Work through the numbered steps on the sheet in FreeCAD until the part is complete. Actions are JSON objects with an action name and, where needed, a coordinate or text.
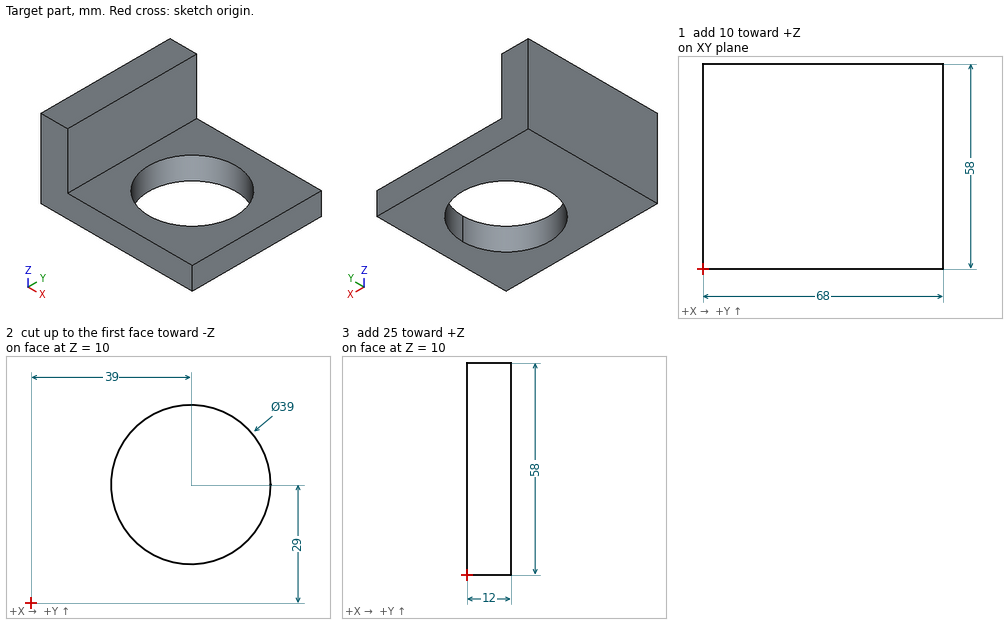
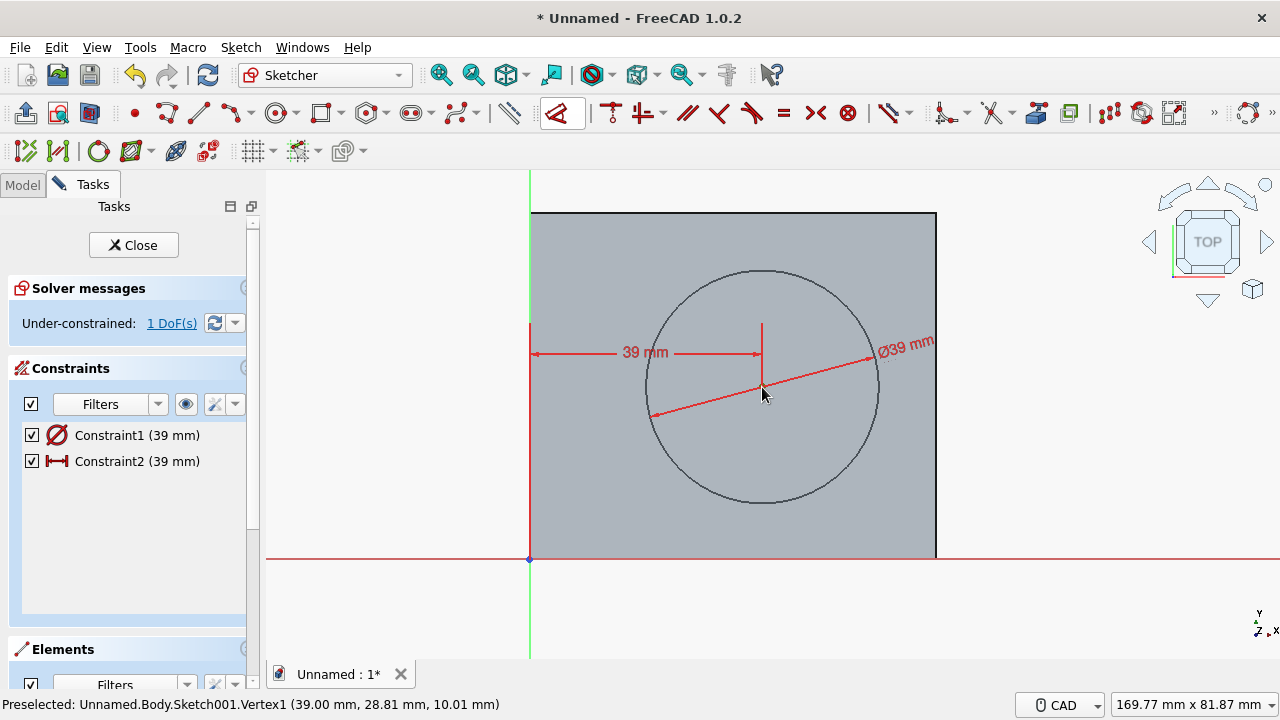
{"action": "key", "text": "i"}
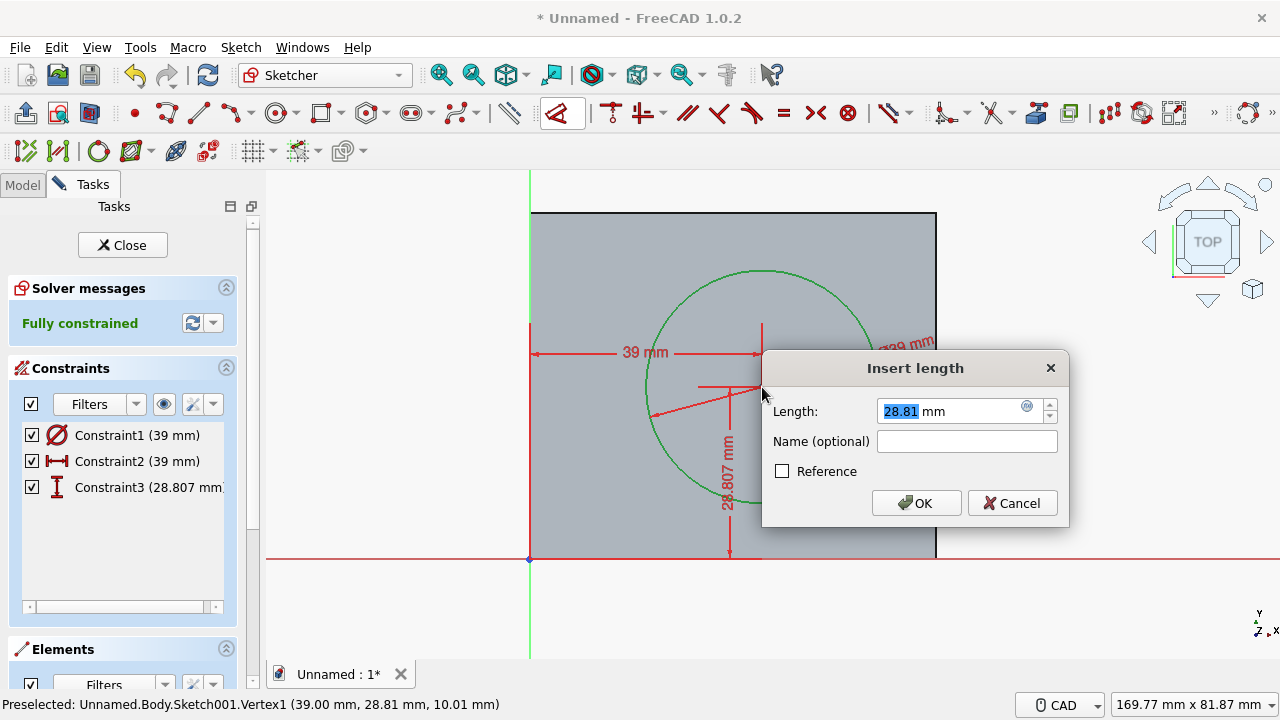
{"action": "type", "text": "29"}
{"action": "key", "text": "Return"}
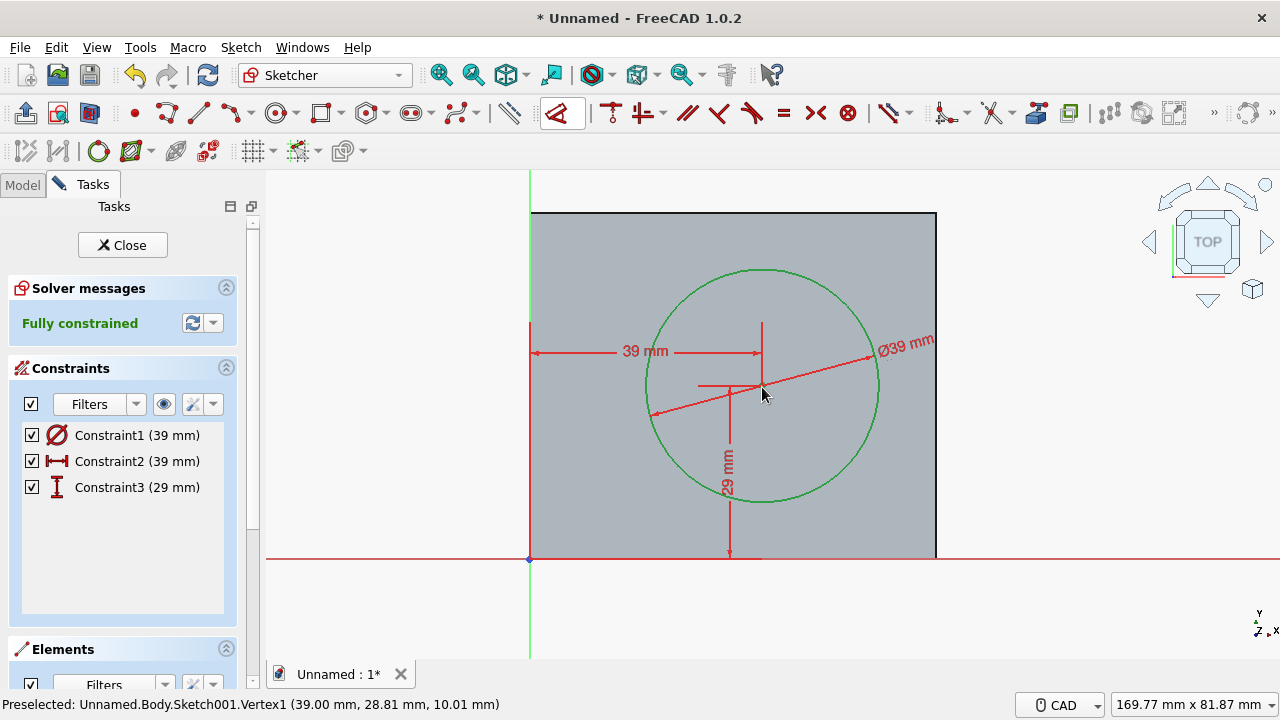
{"action": "left_click", "coordinate": [123, 245]}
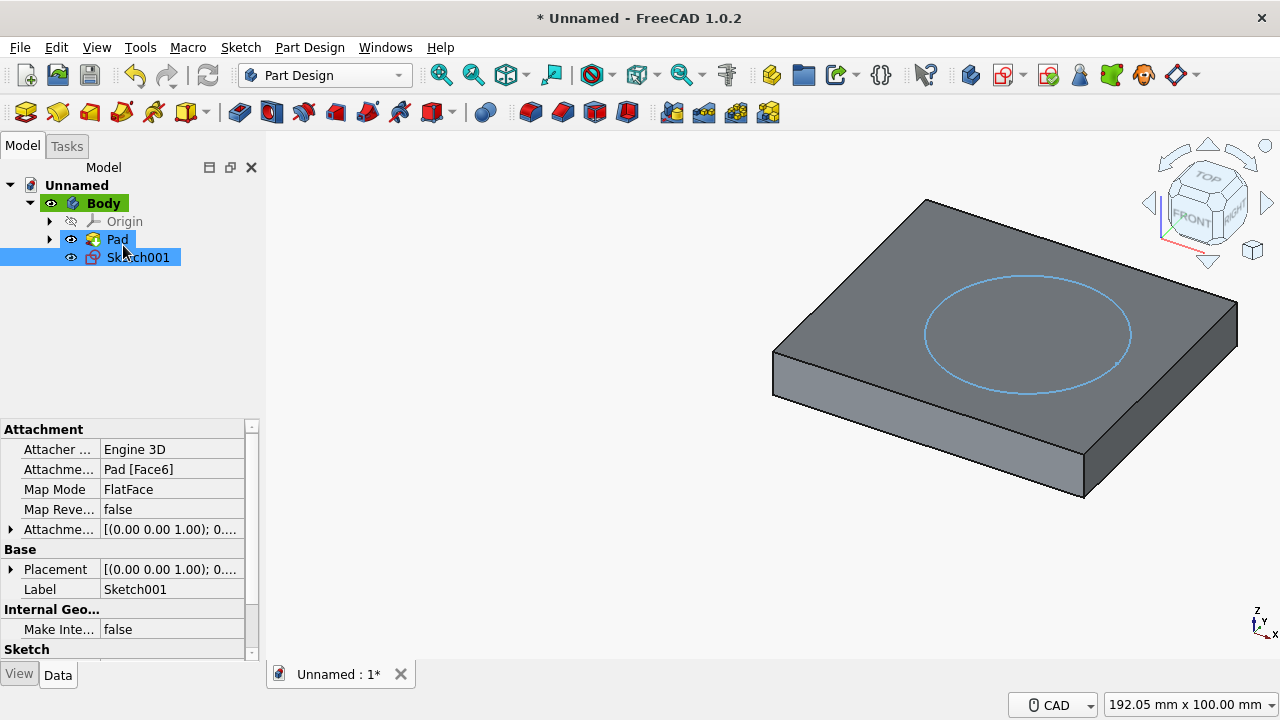
{"action": "left_click", "coordinate": [240, 112]}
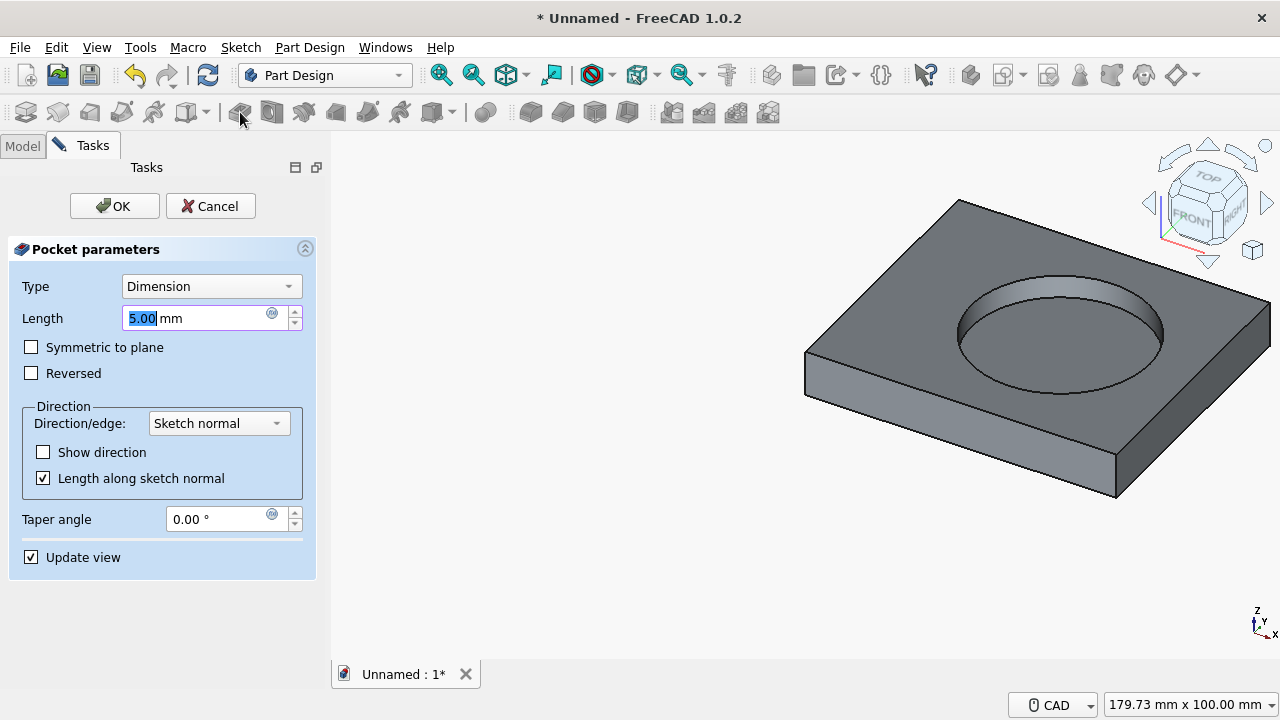
{"action": "left_click", "coordinate": [212, 286]}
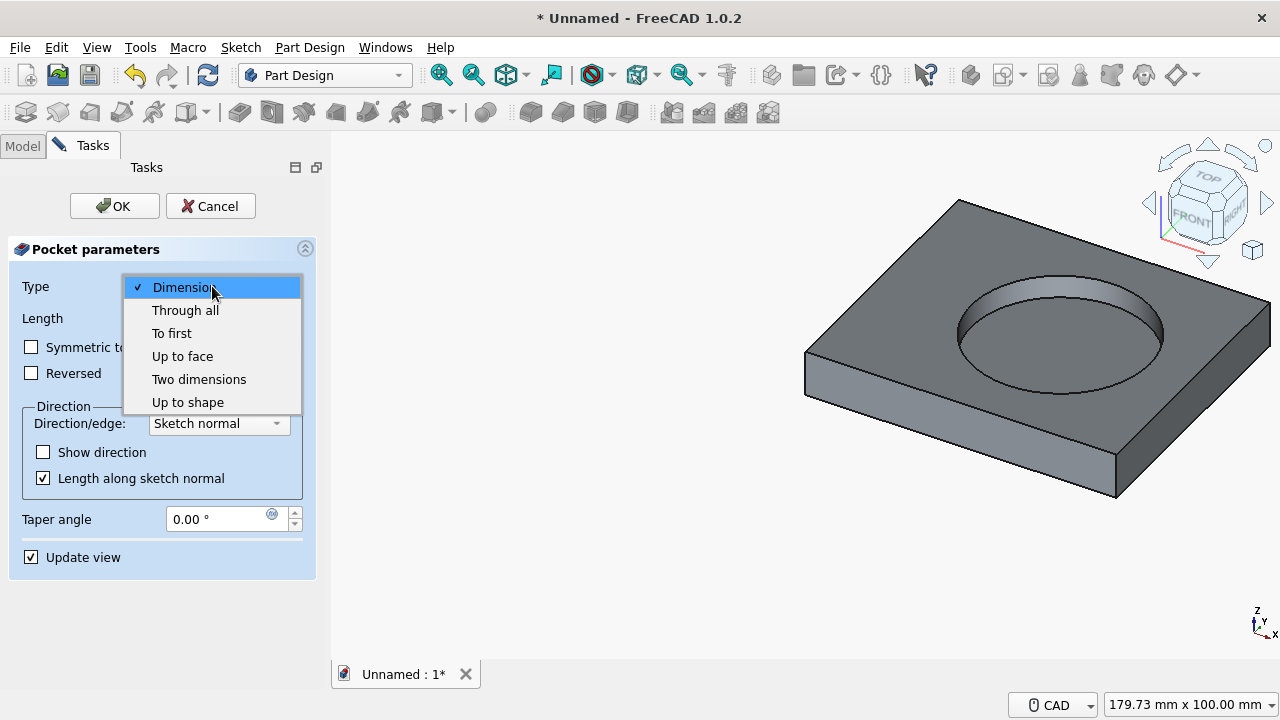
{"action": "left_click", "coordinate": [212, 334]}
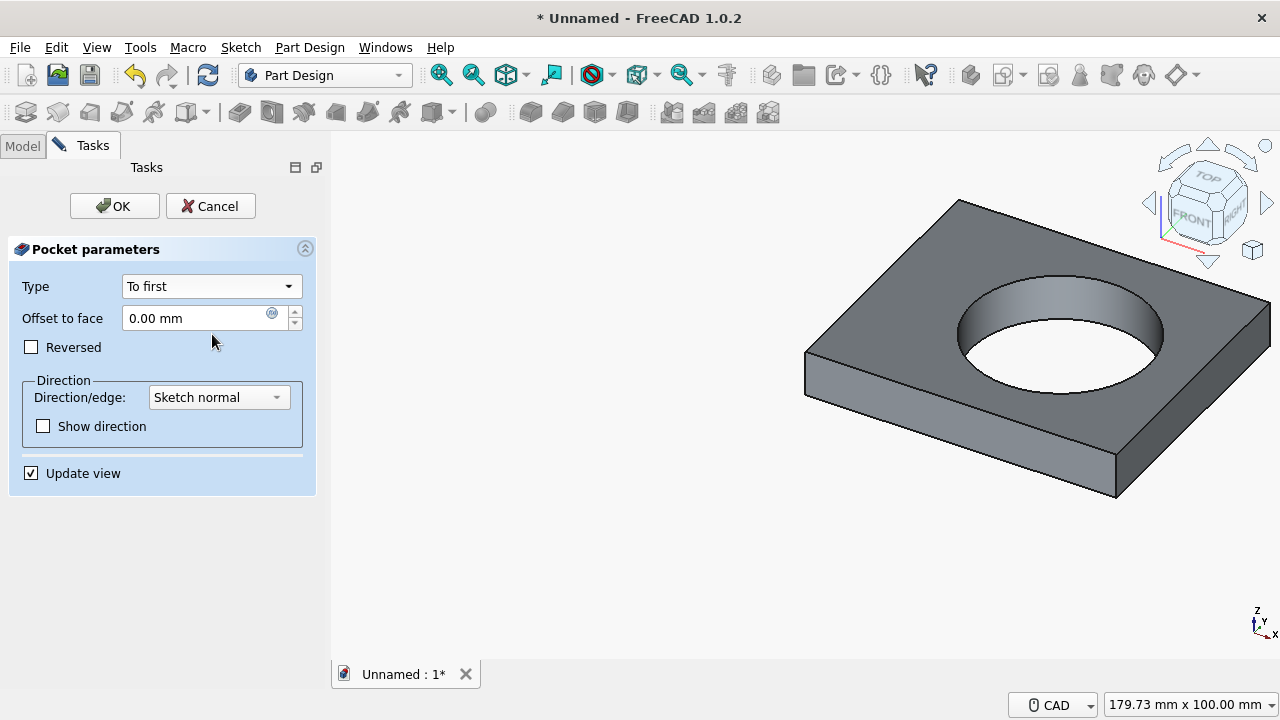
{"action": "left_click", "coordinate": [115, 206]}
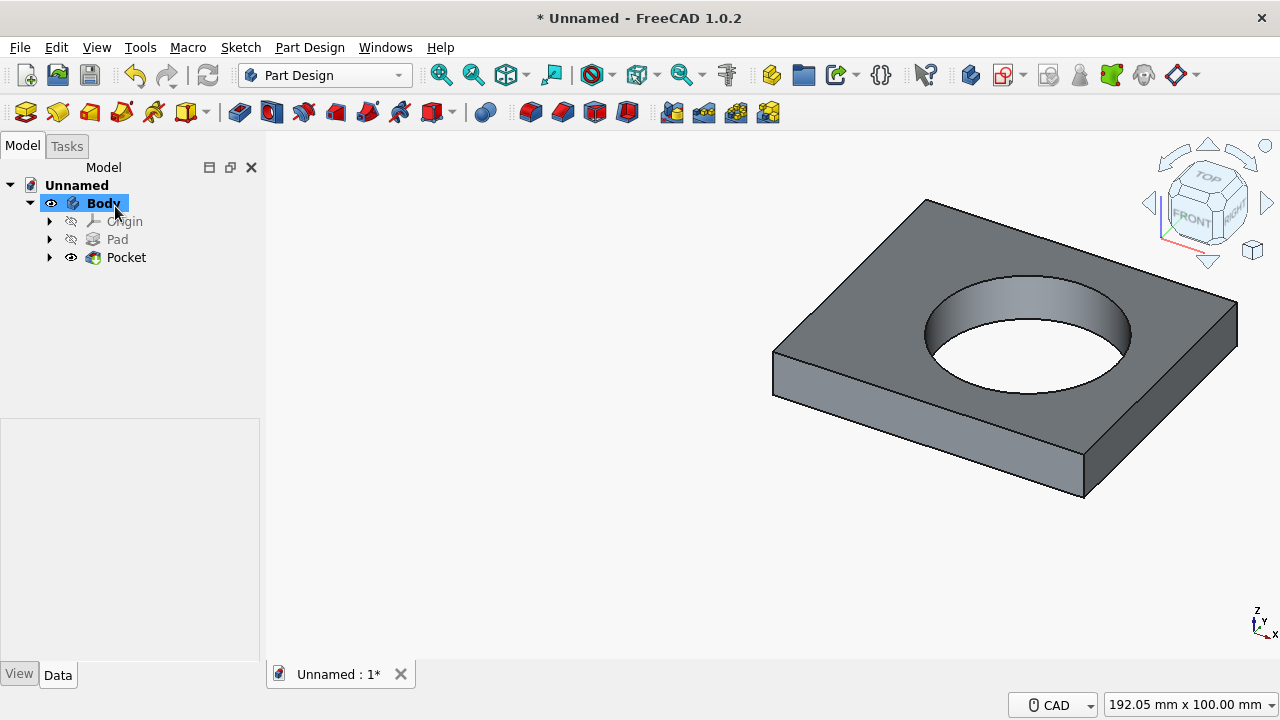
{"action": "left_click", "coordinate": [872, 340]}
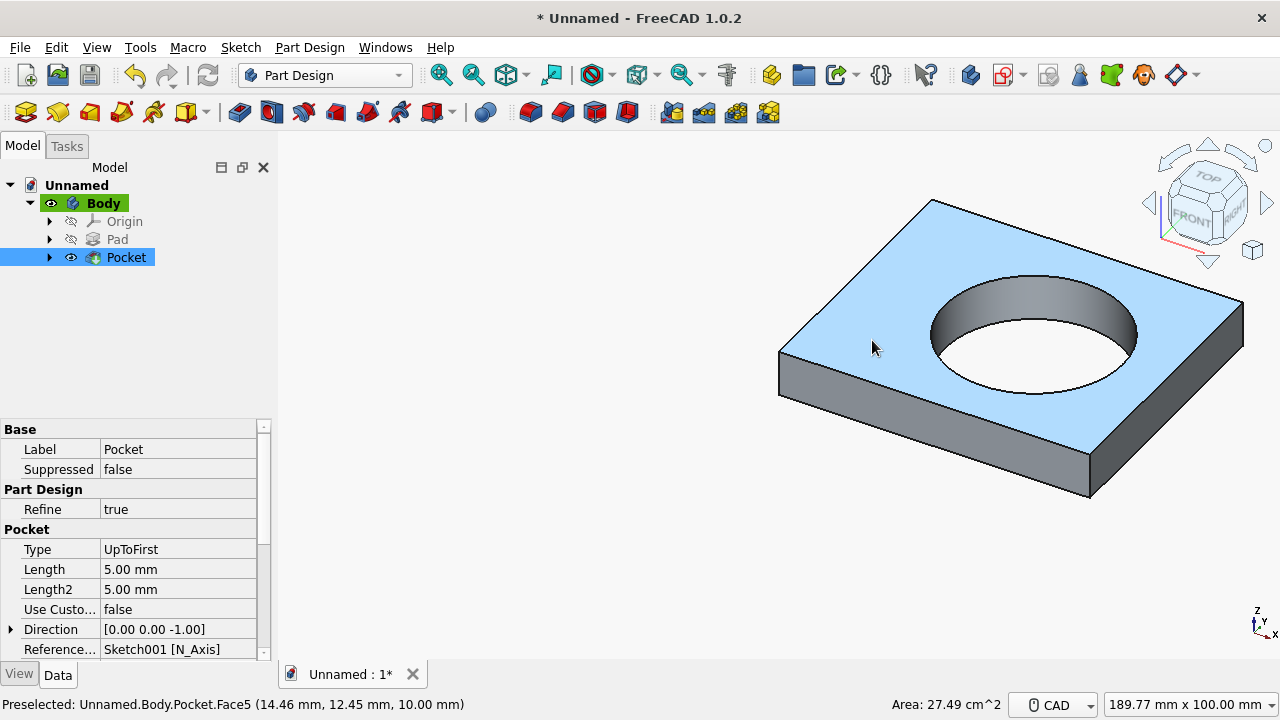
{"action": "left_click", "coordinate": [1004, 76]}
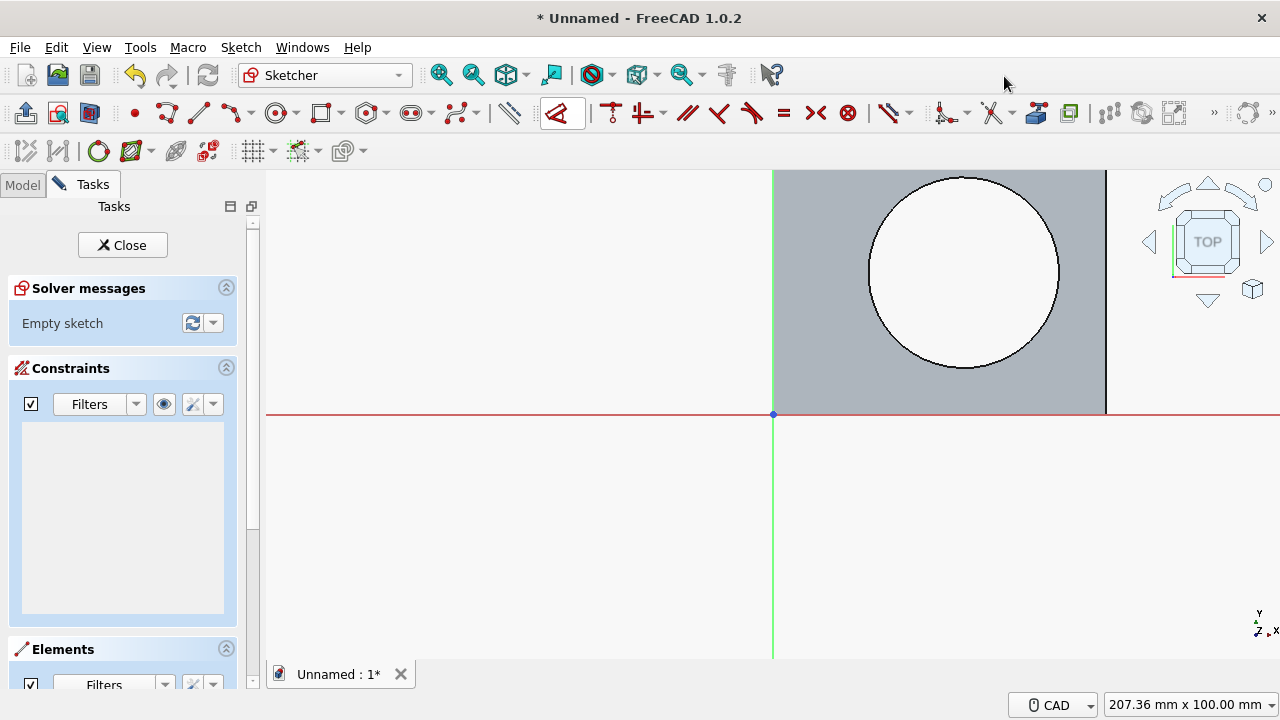
{"action": "scroll", "coordinate": [506, 631], "scroll_direction": "down", "scroll_amount": 2}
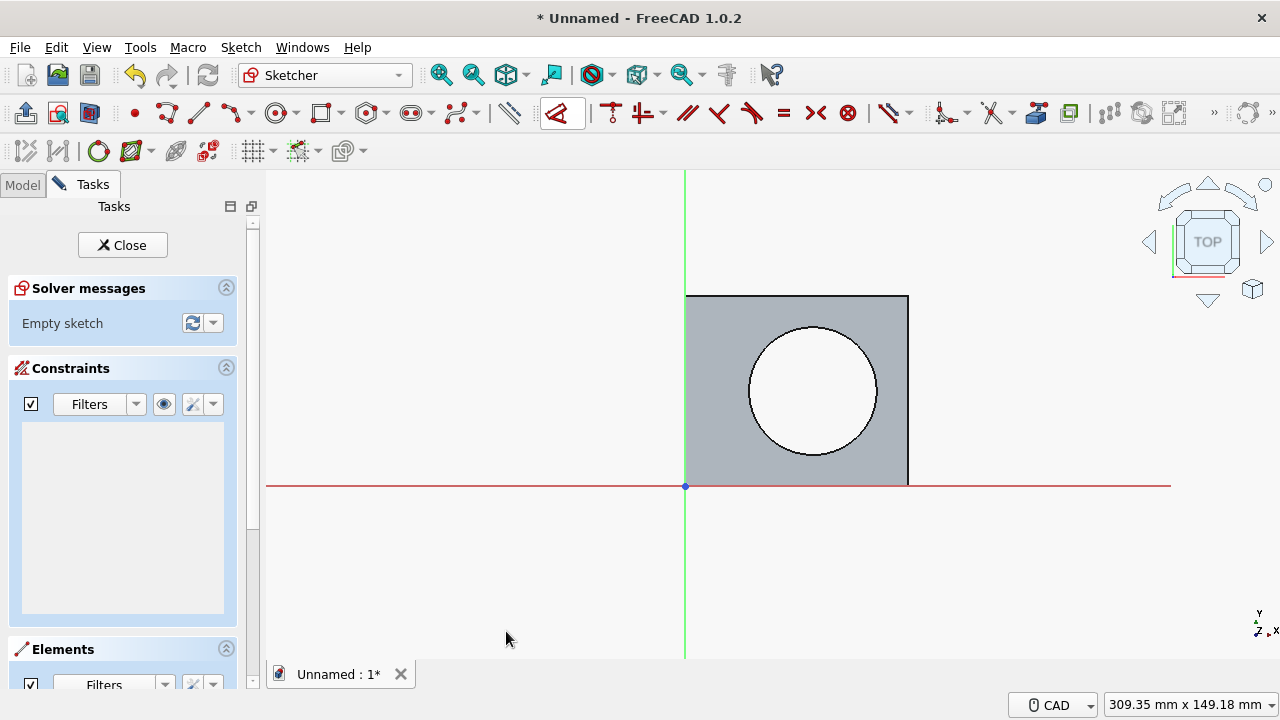
{"action": "scroll", "coordinate": [705, 344], "scroll_direction": "up", "scroll_amount": 2}